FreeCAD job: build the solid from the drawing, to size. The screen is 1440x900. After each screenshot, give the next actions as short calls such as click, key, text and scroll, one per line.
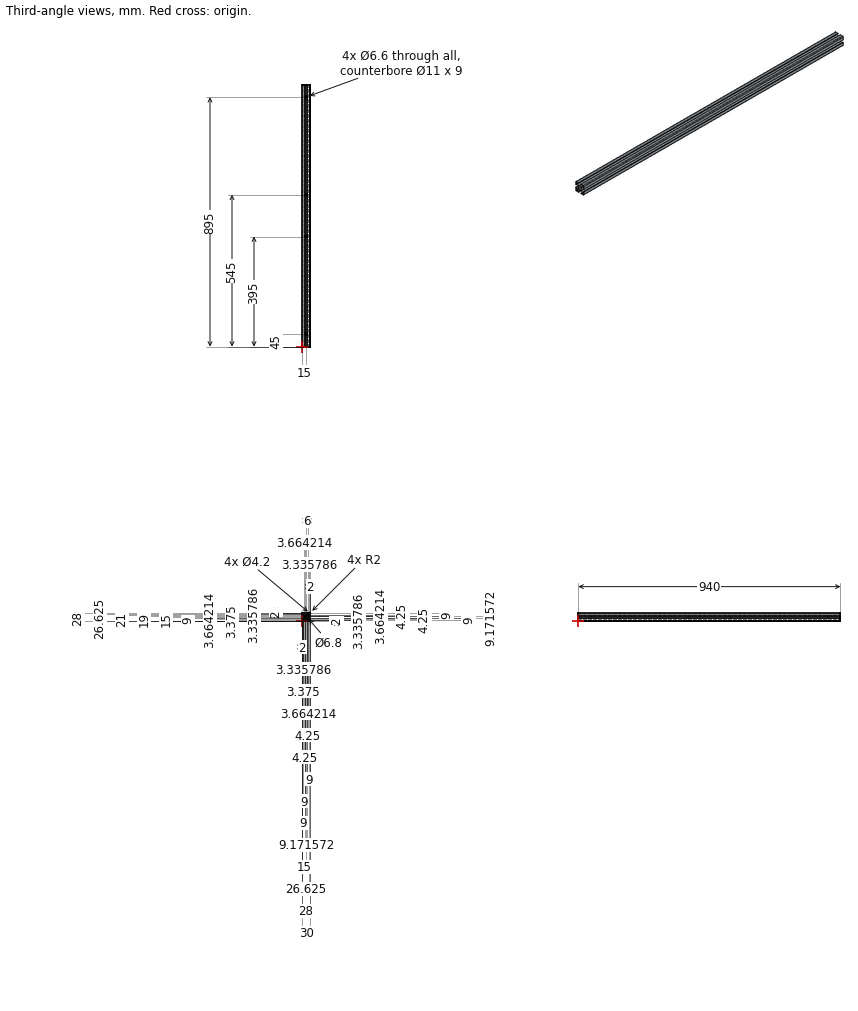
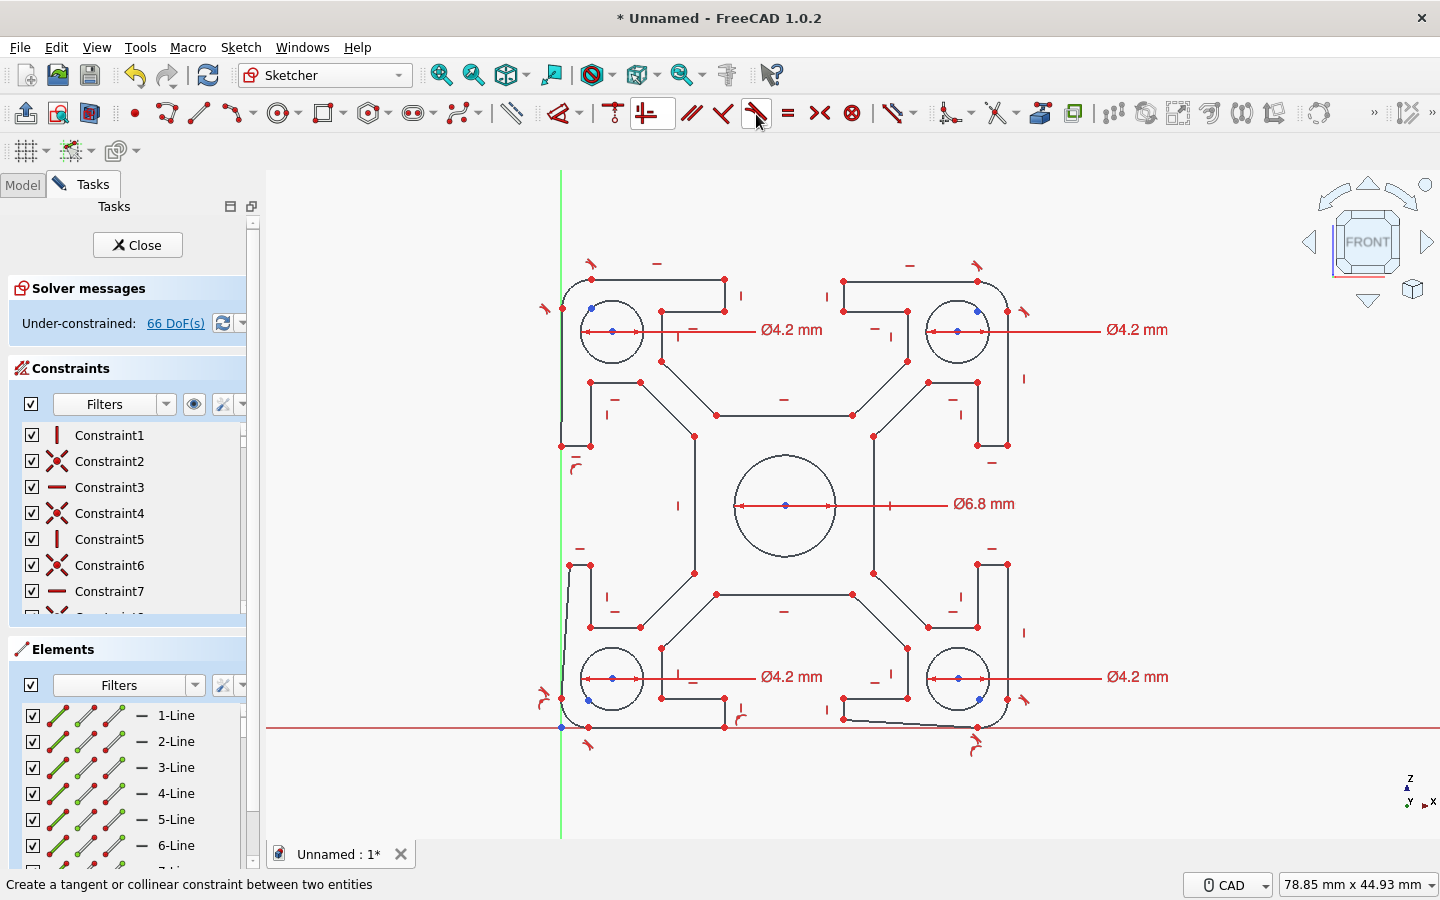
click(938, 726)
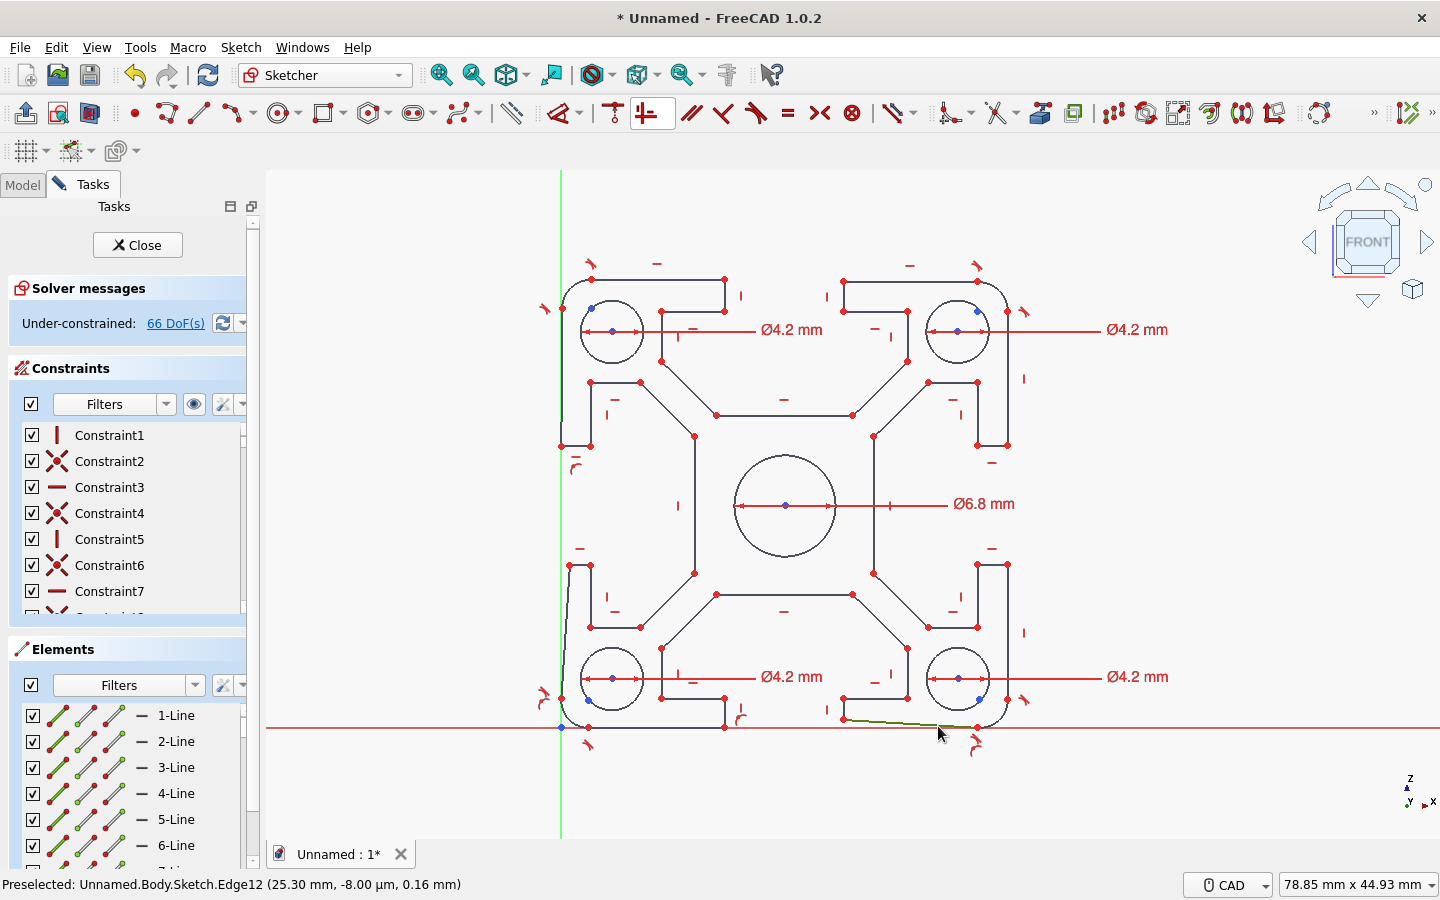
key(h)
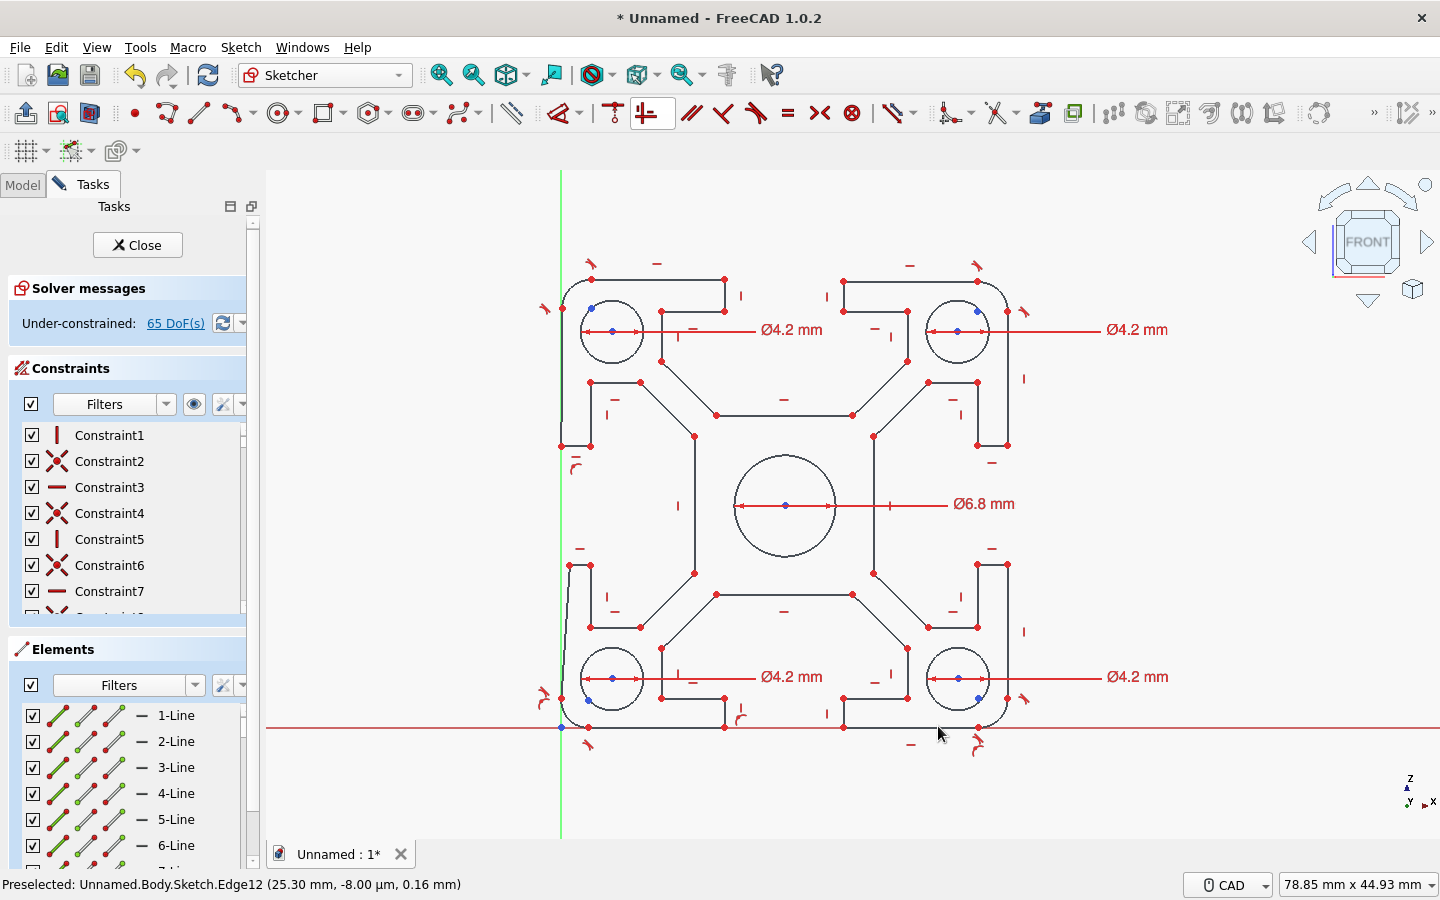
click(684, 728)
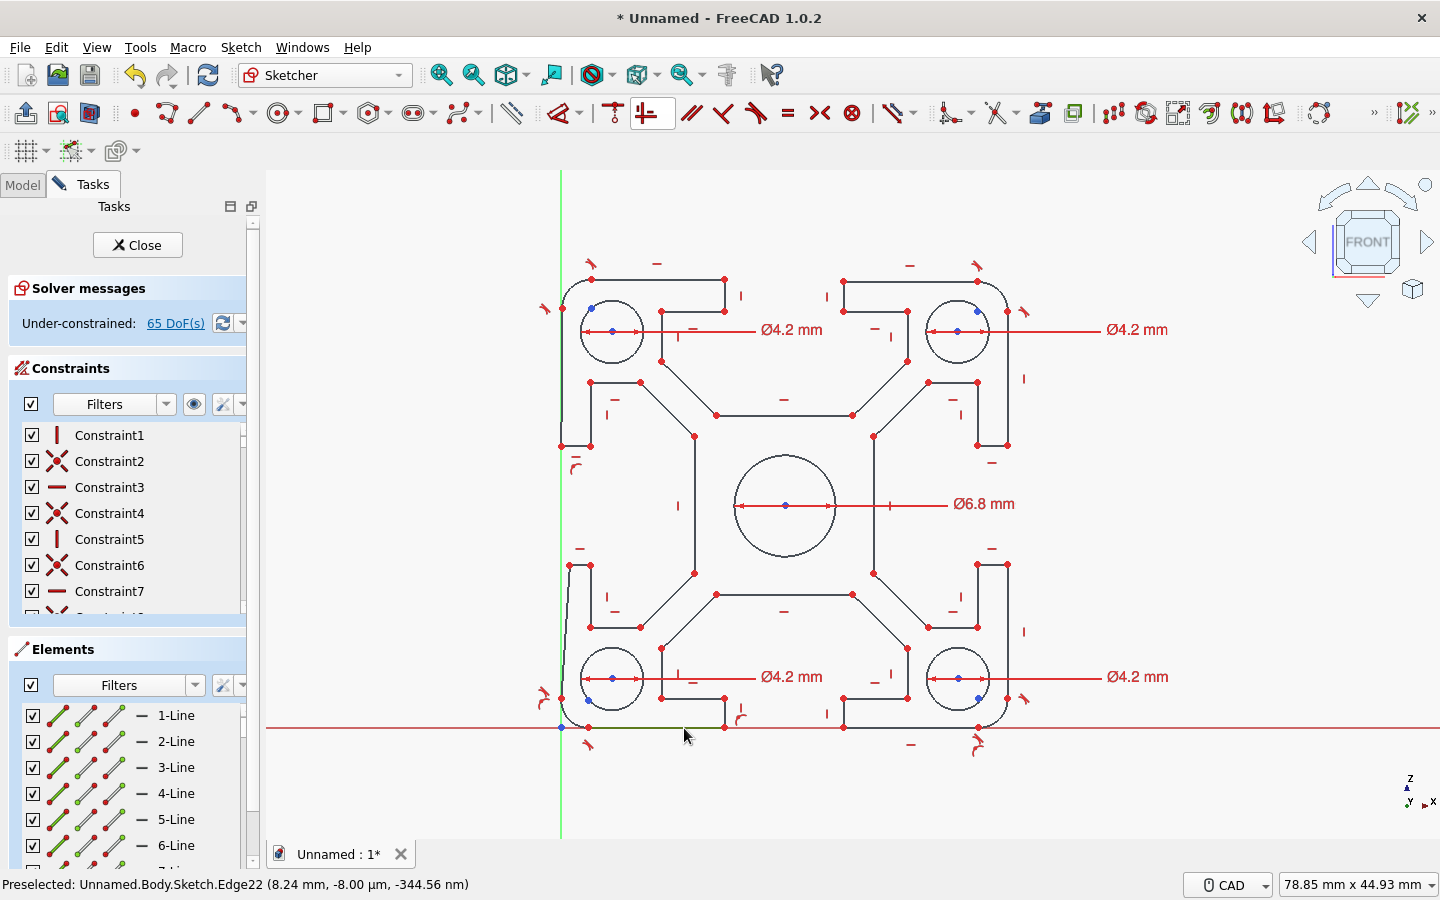
key(h)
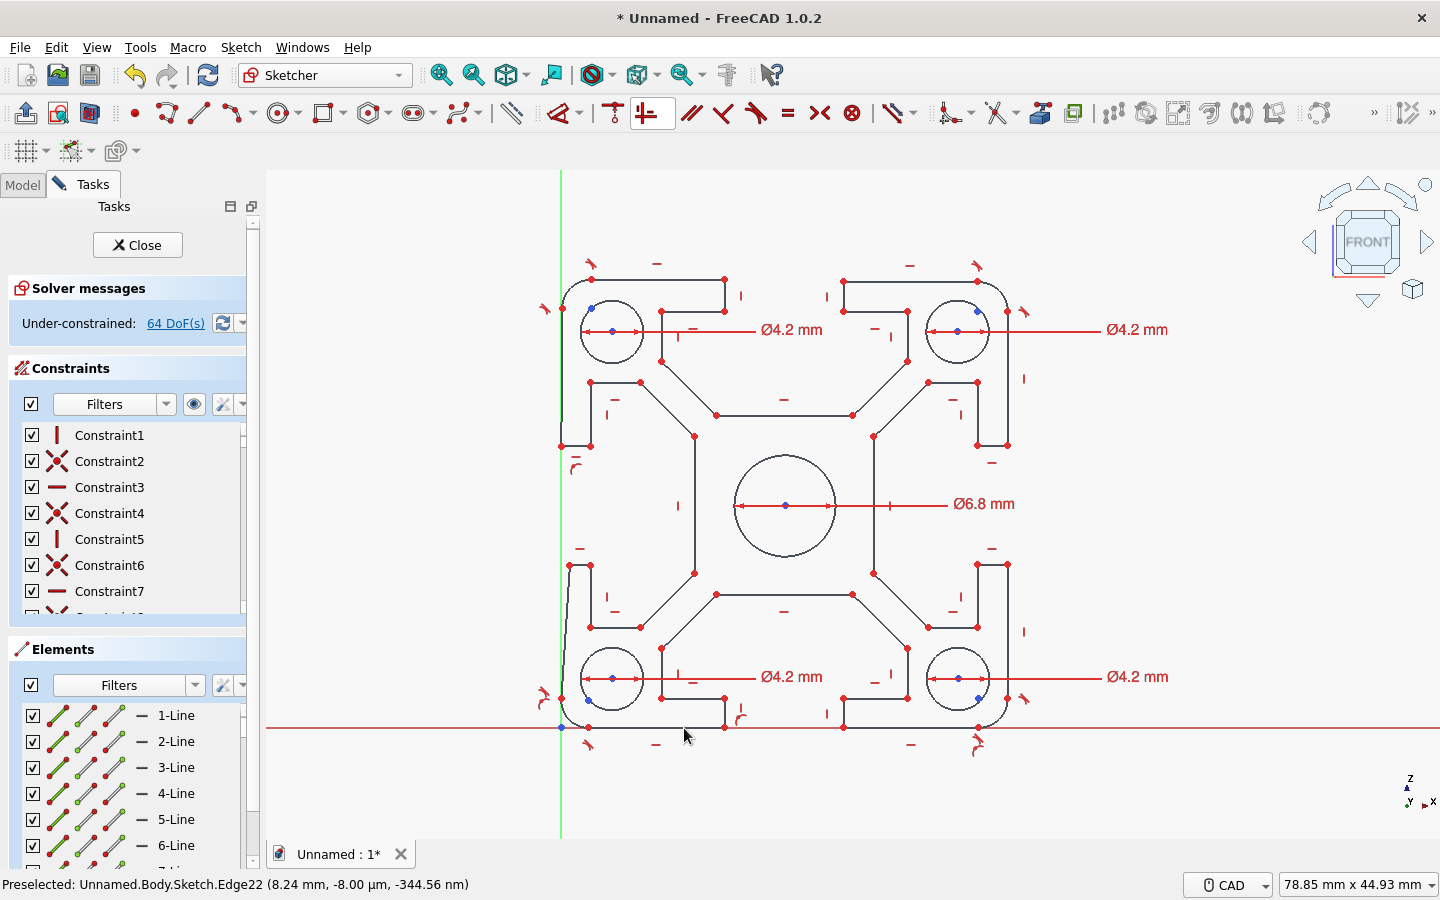
click(564, 659)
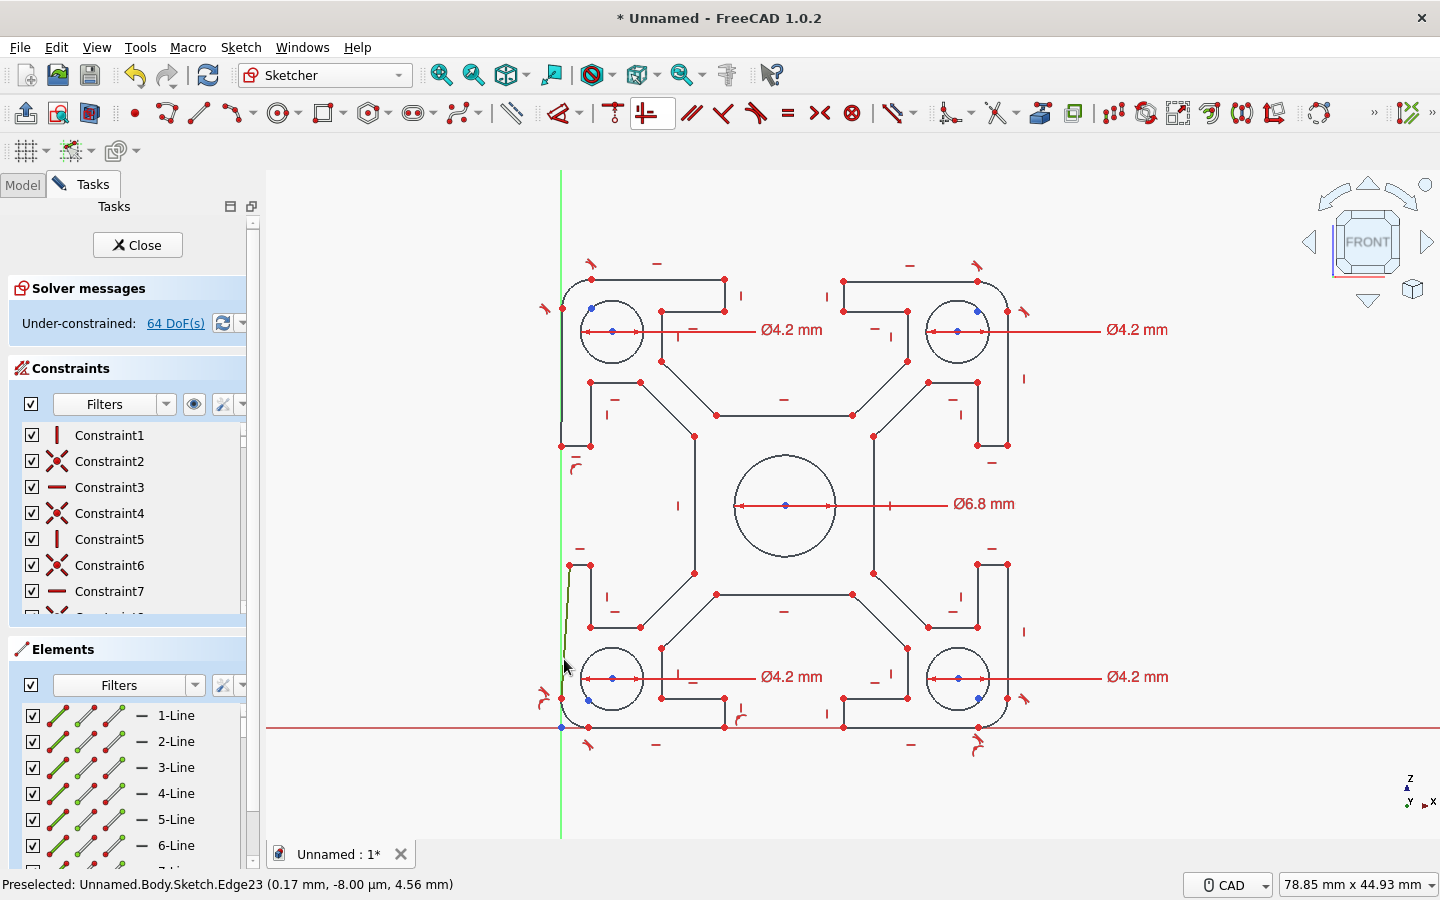
key(v)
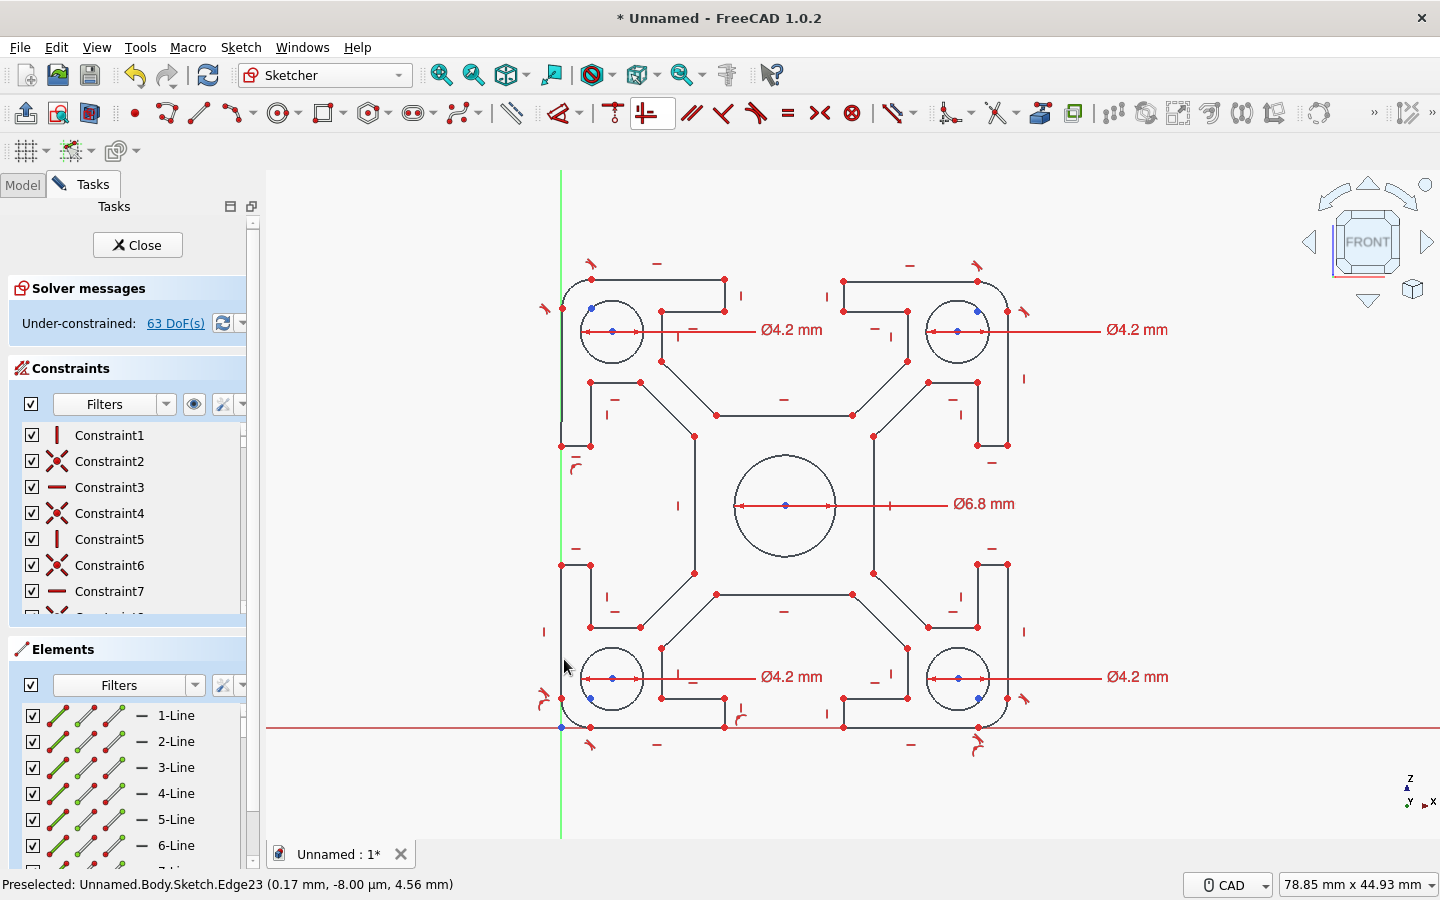
click(562, 405)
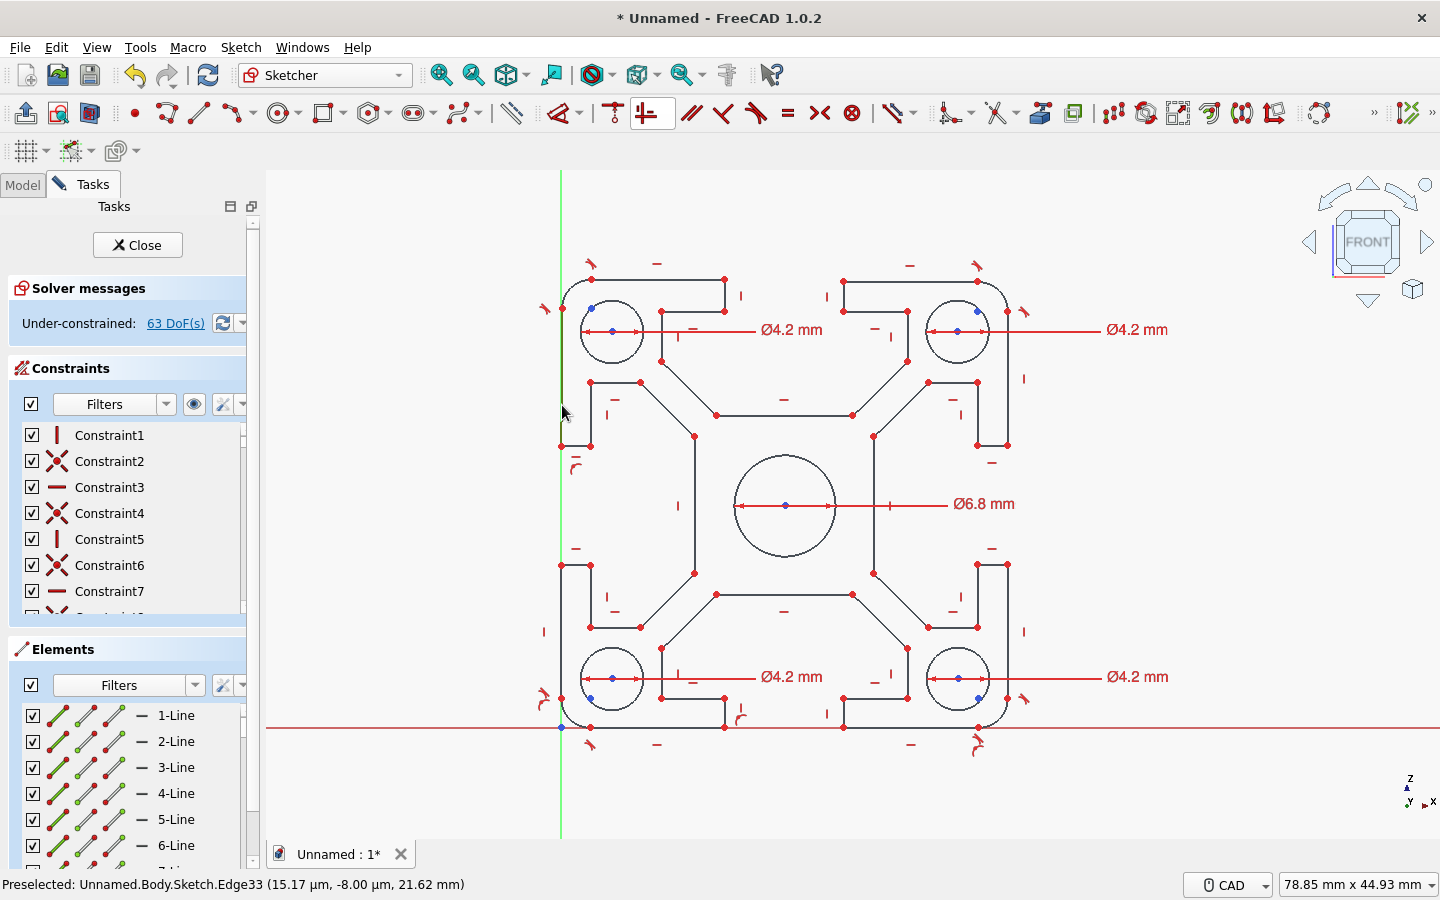
key(v)